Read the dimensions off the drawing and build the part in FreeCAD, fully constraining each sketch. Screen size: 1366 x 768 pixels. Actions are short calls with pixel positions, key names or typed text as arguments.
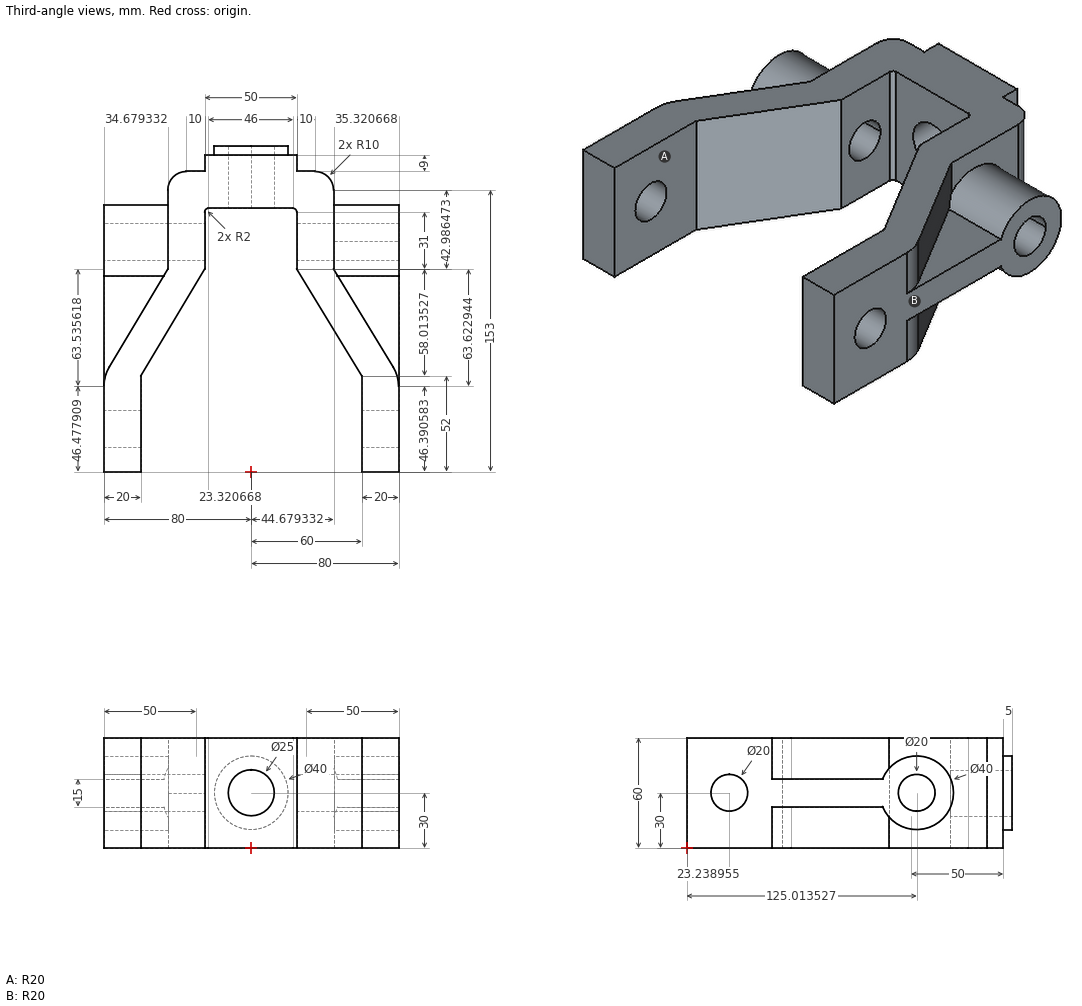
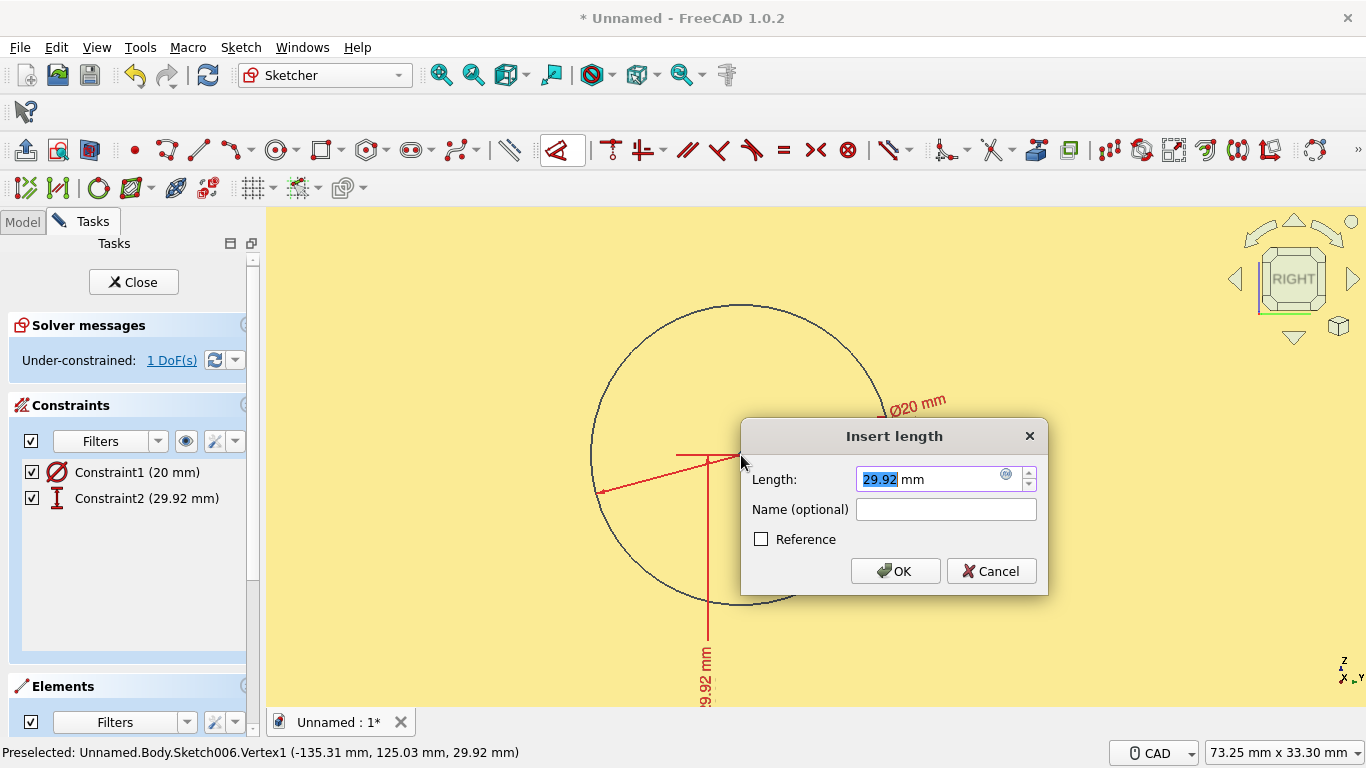
text(30)
key(Return)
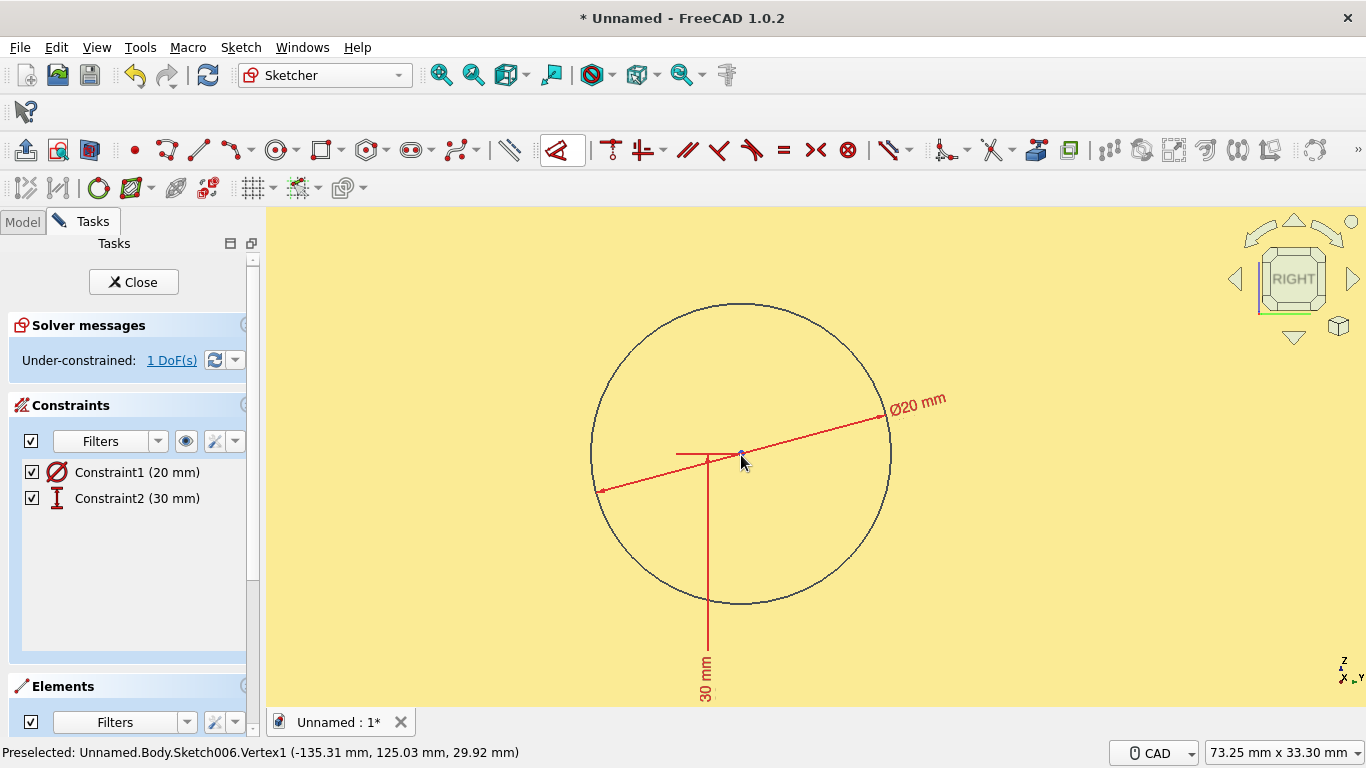
click(741, 454)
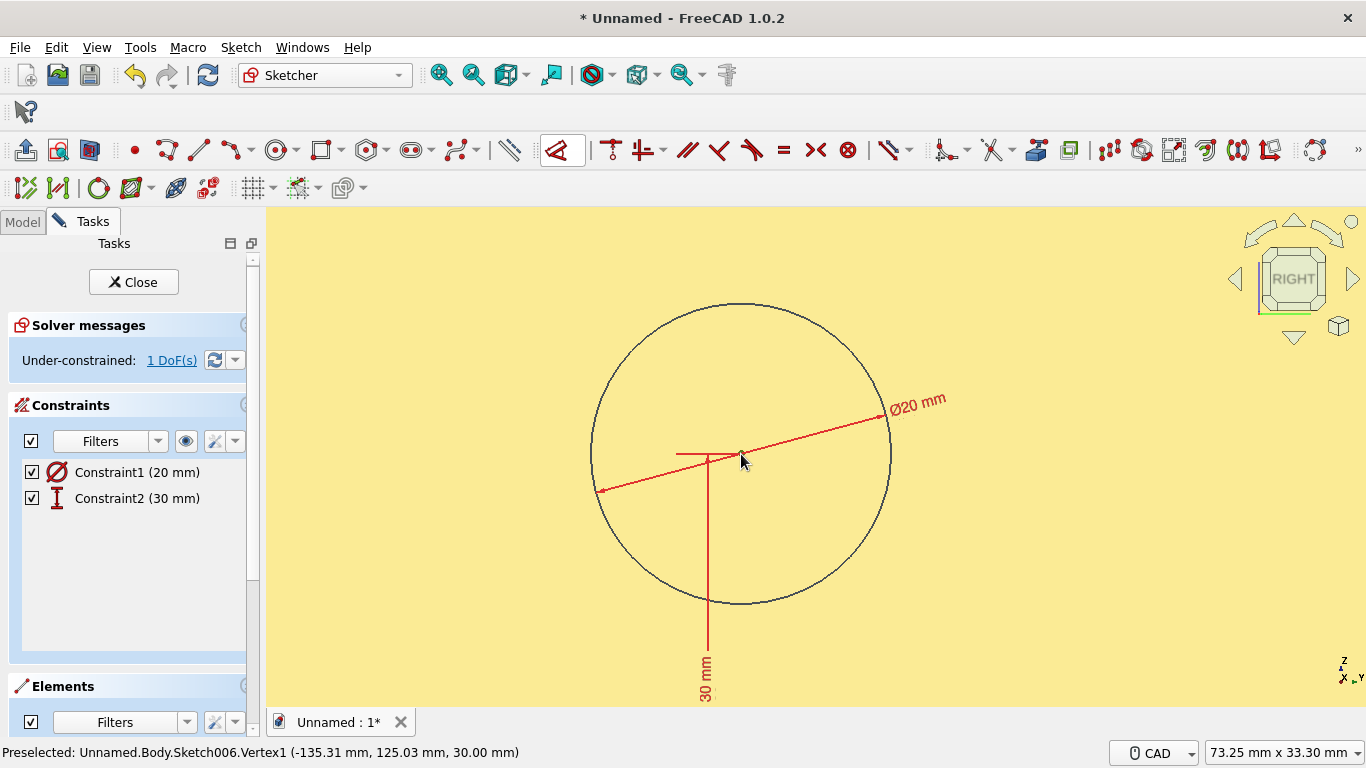
click(580, 150)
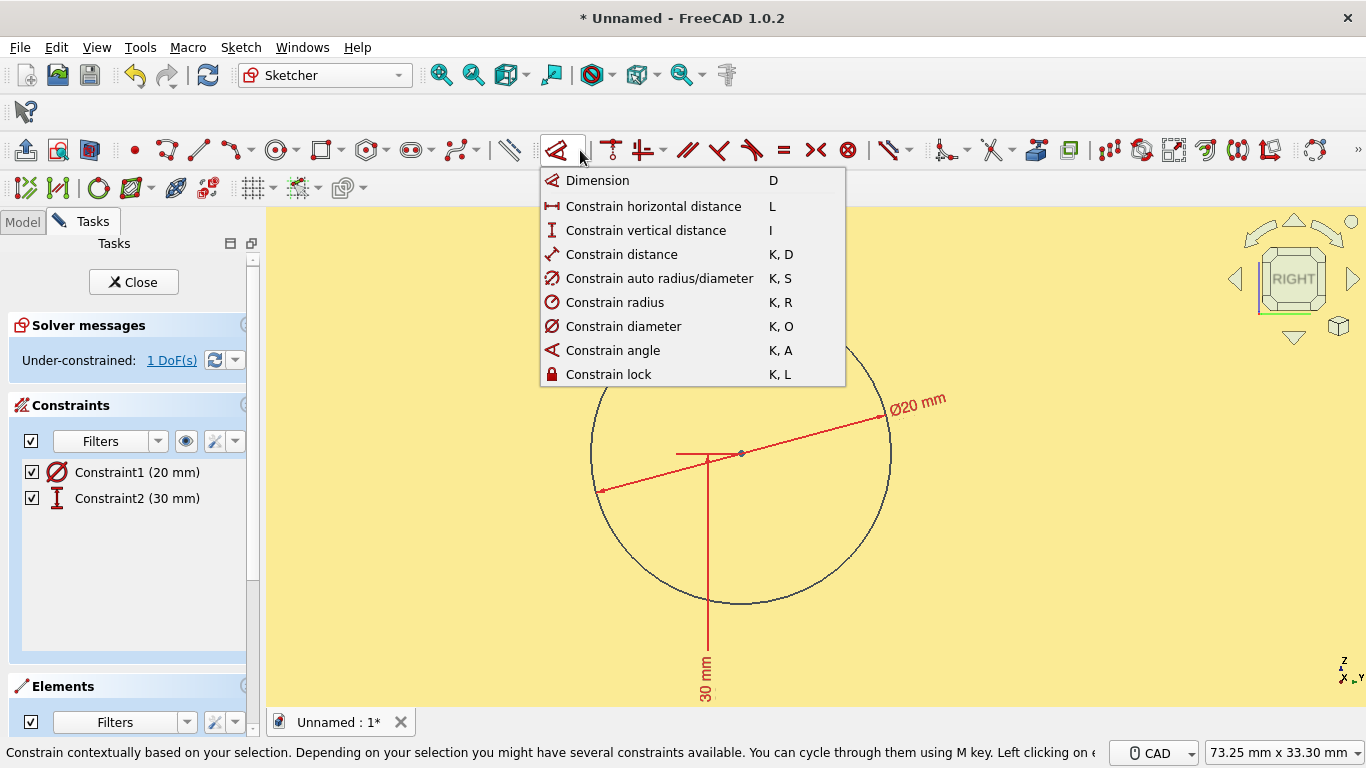
click(693, 206)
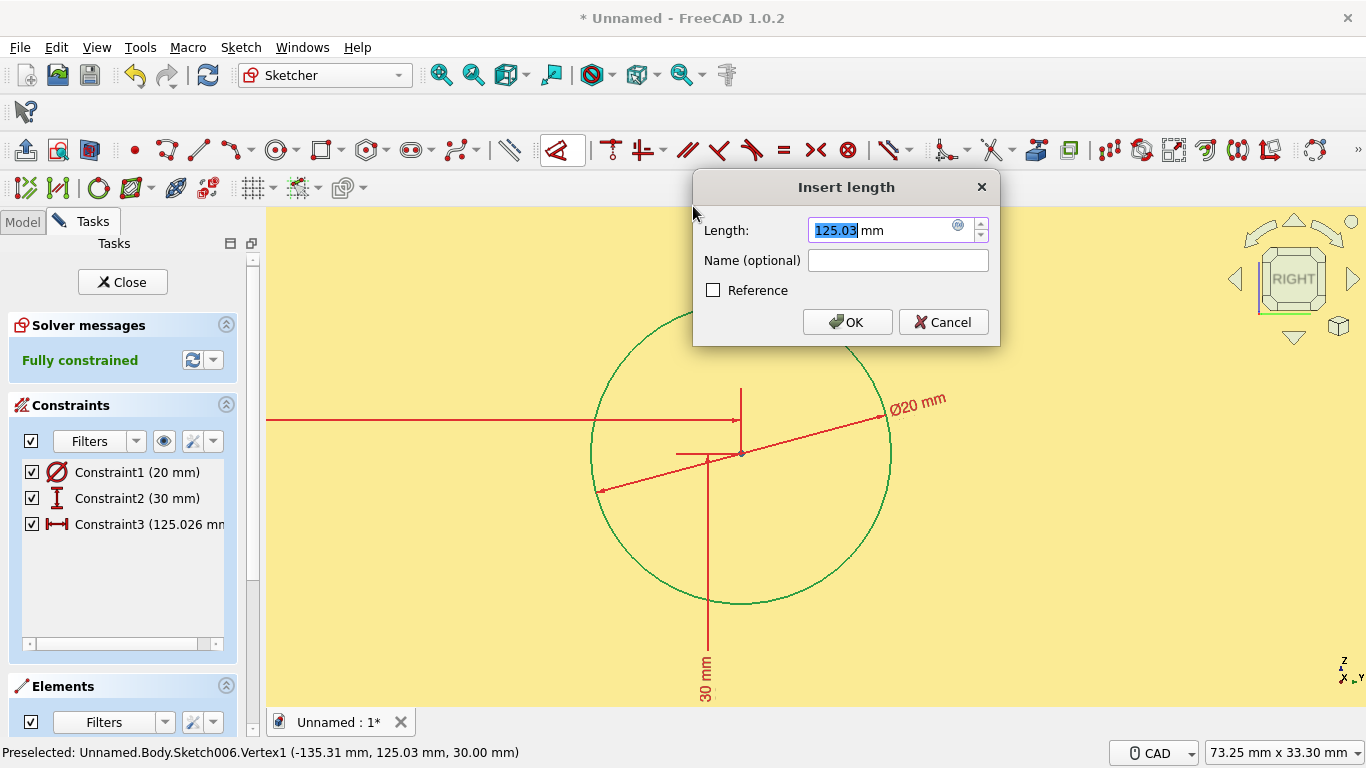
text(125.013527)
key(Return)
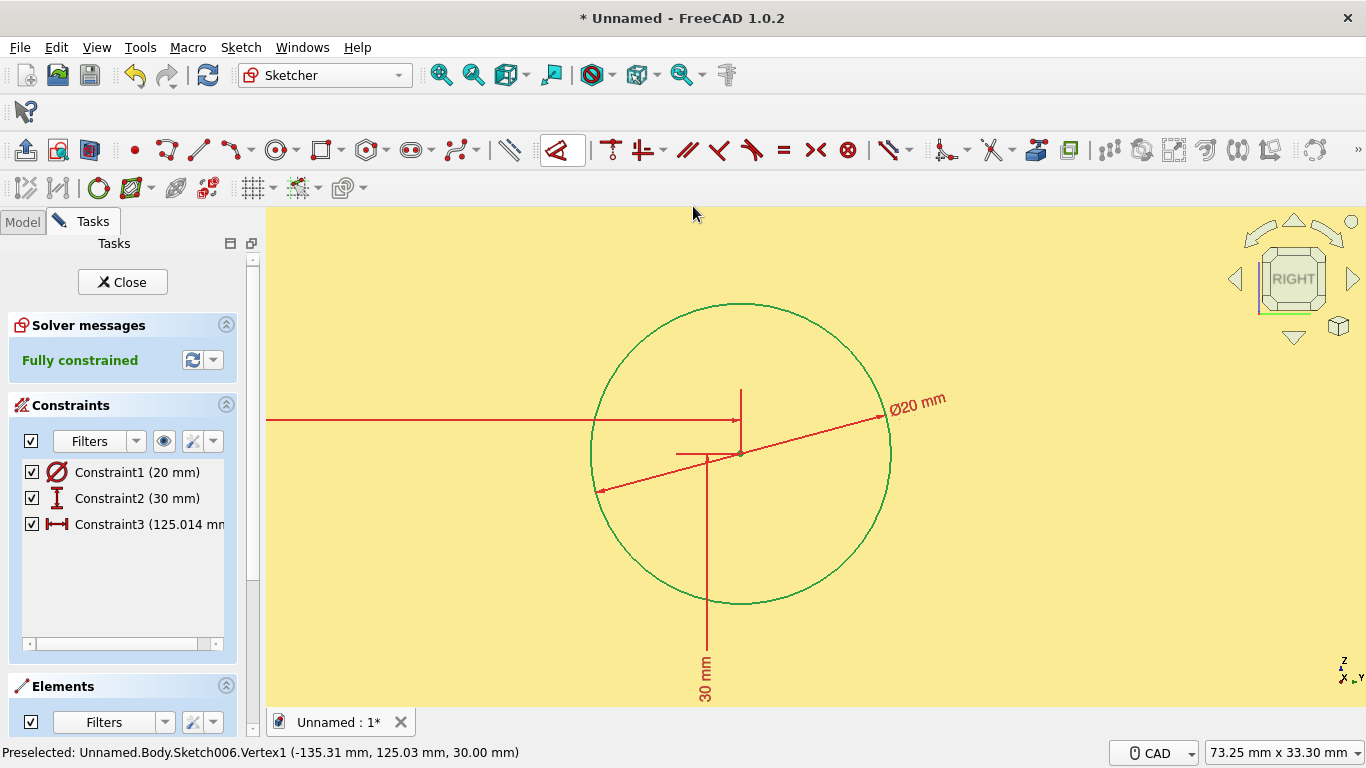
click(123, 282)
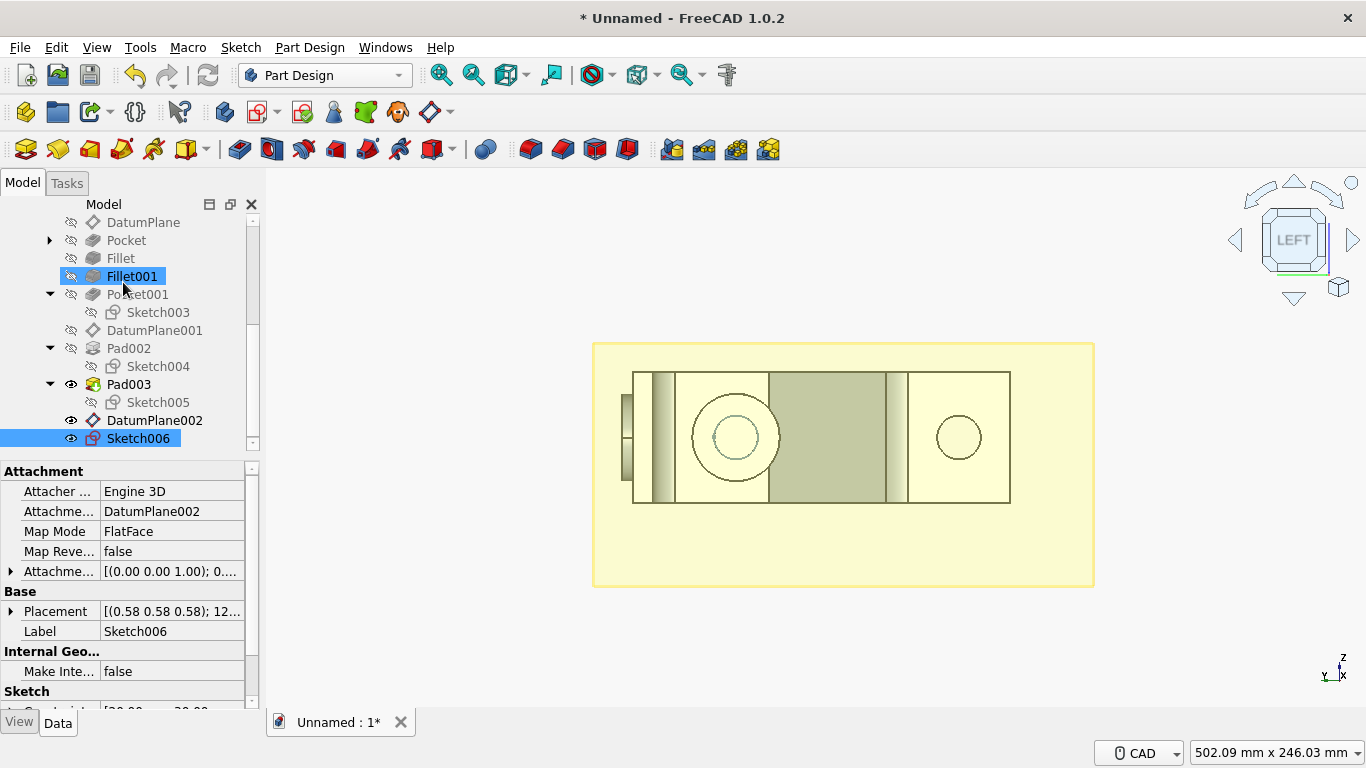
click(240, 150)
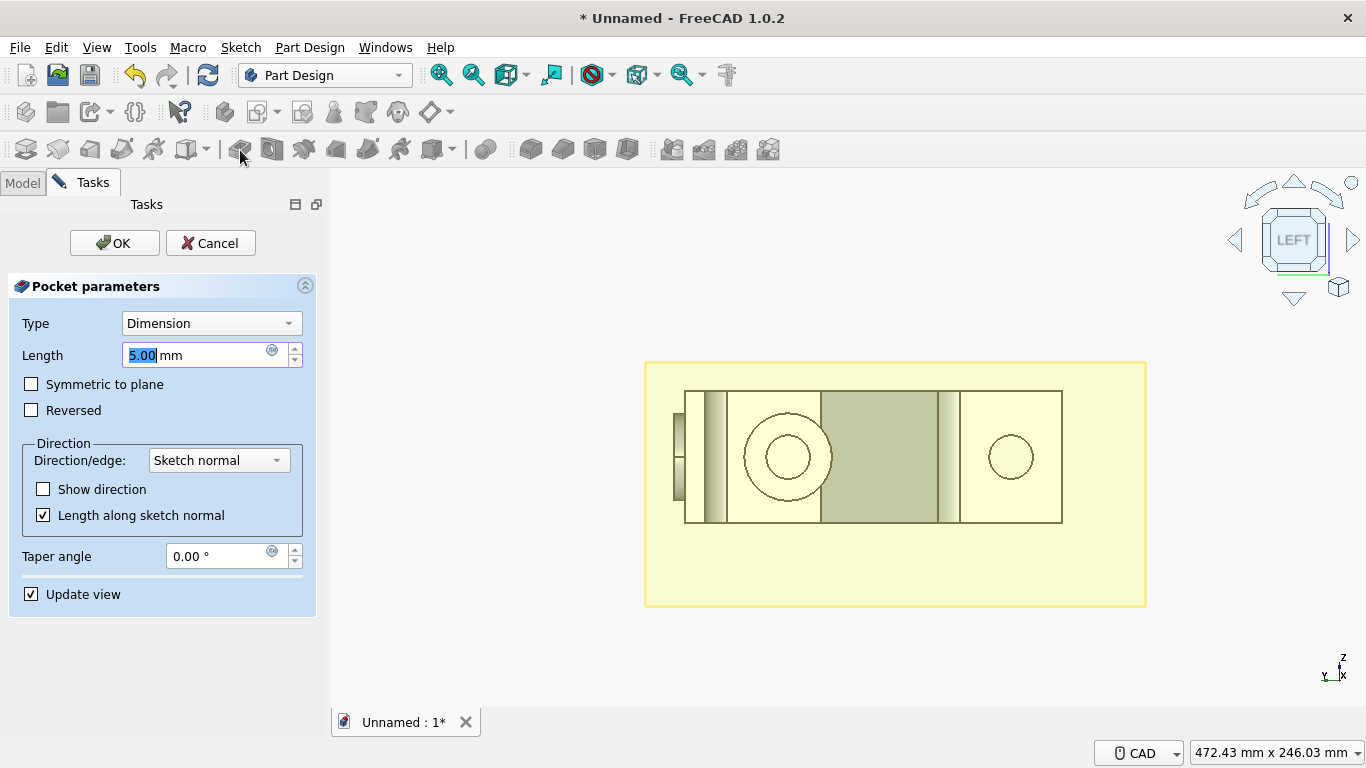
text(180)
key(Tab)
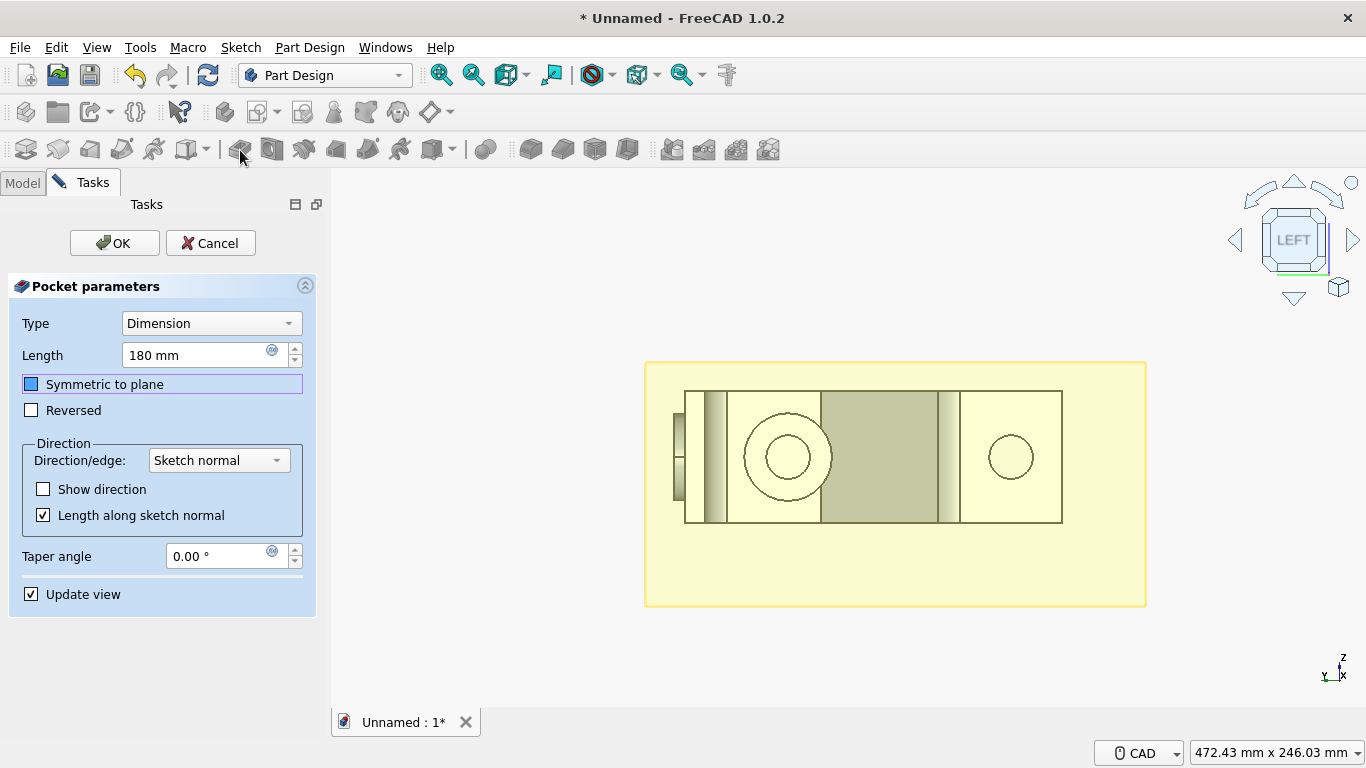
click(30, 410)